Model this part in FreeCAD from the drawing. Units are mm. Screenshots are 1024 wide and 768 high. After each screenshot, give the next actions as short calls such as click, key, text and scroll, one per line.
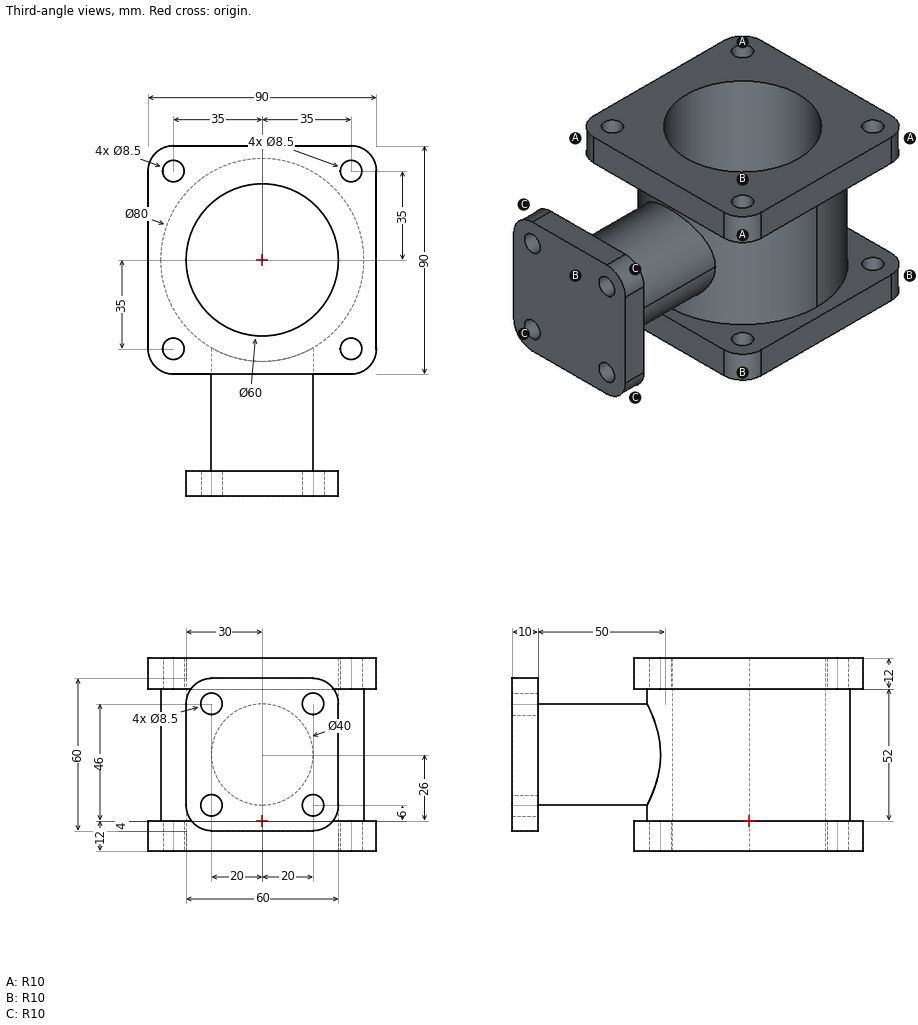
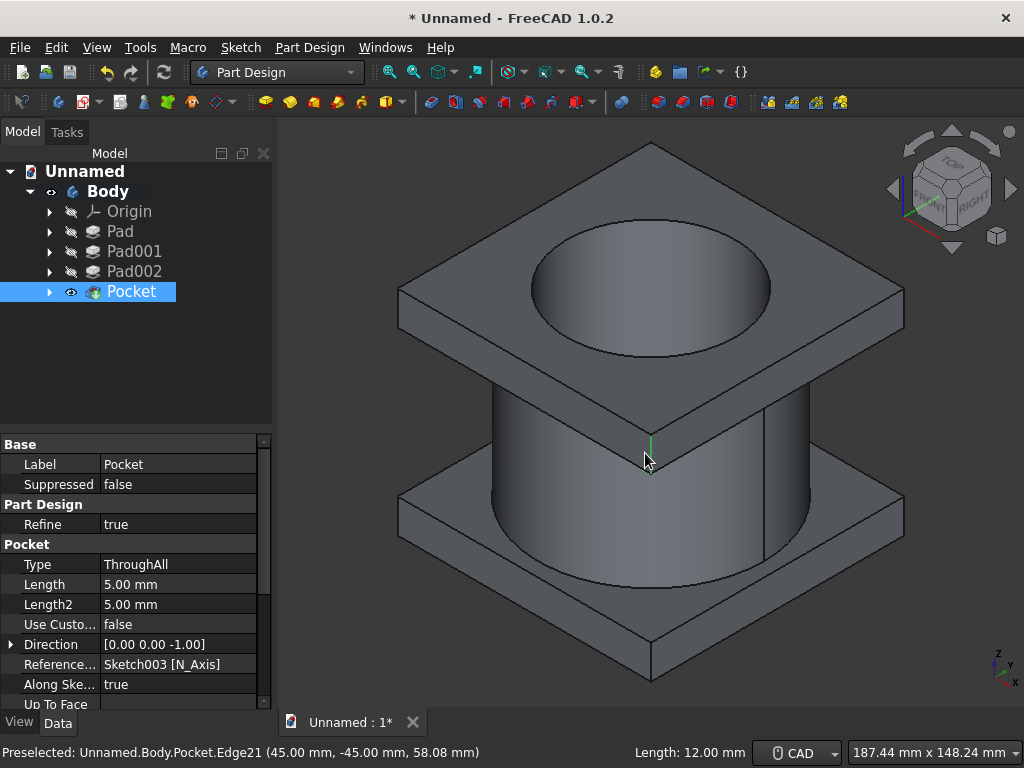
key(1)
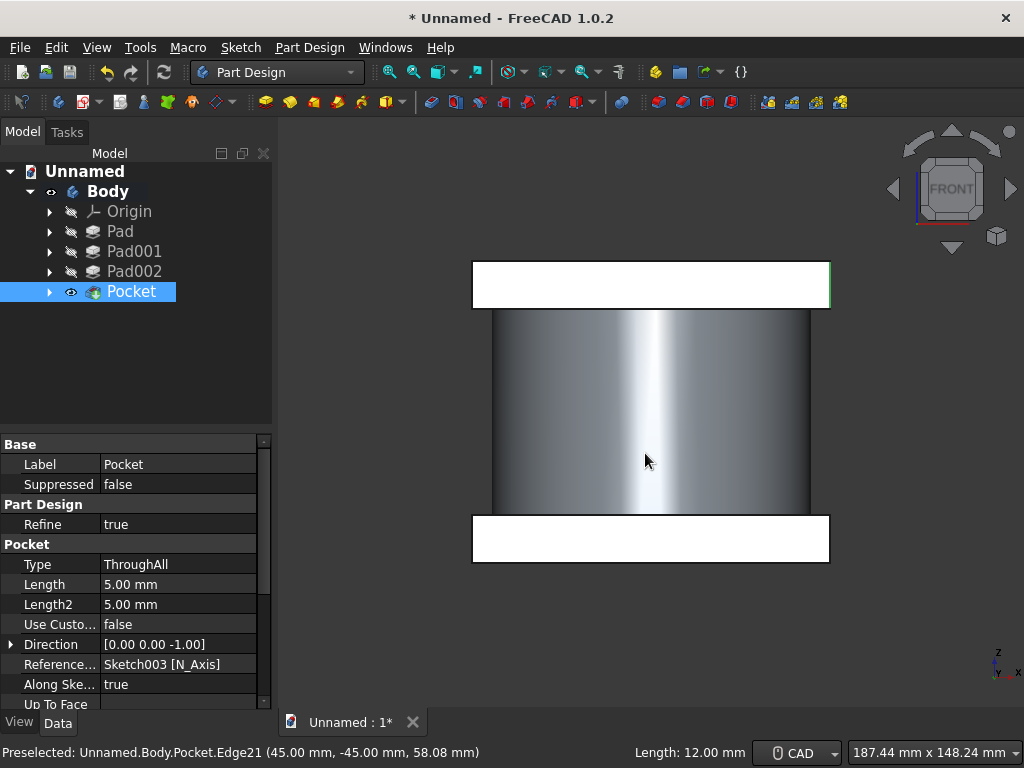
click(472, 284, ctrl)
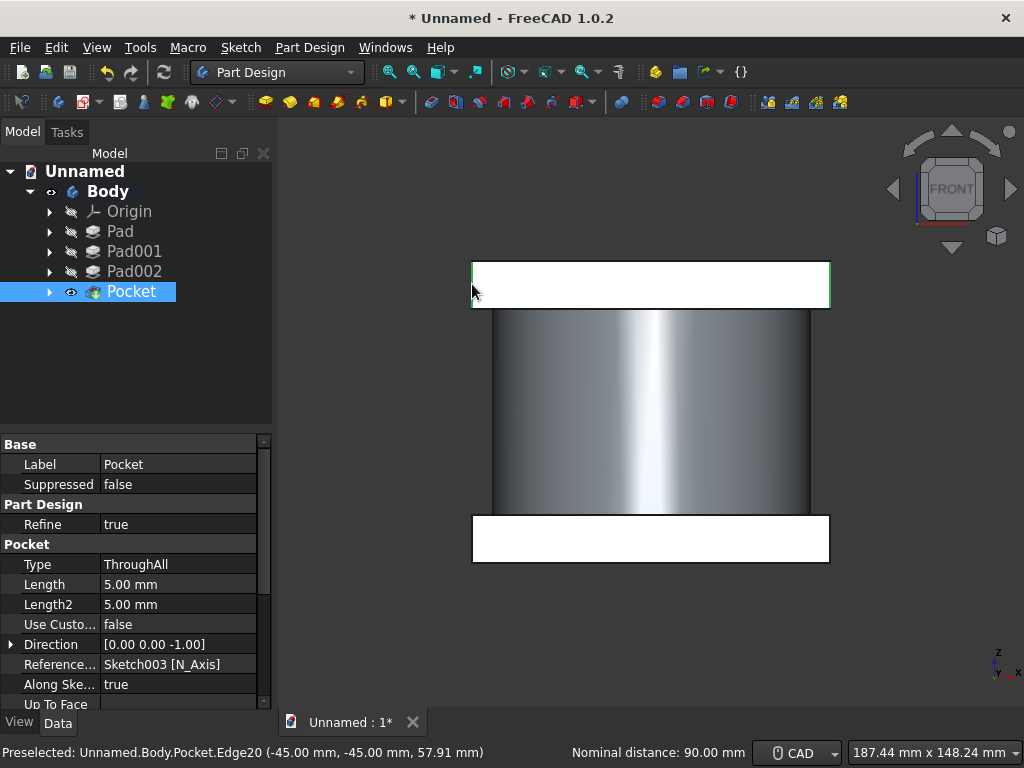
key(3)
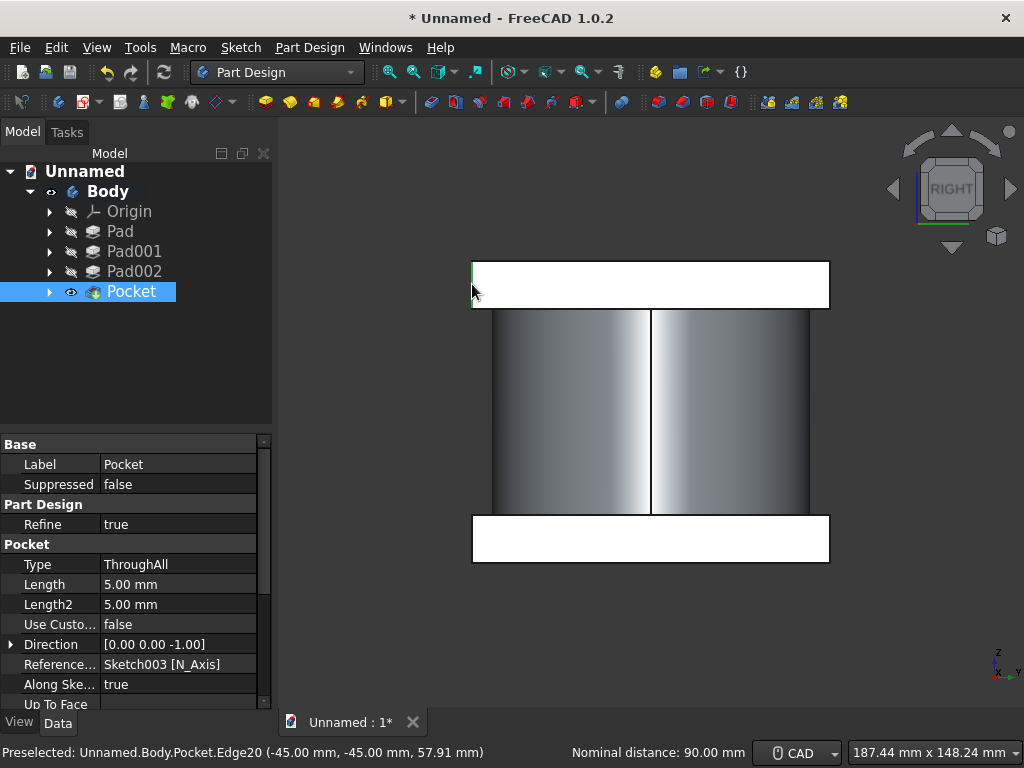
click(830, 284, ctrl)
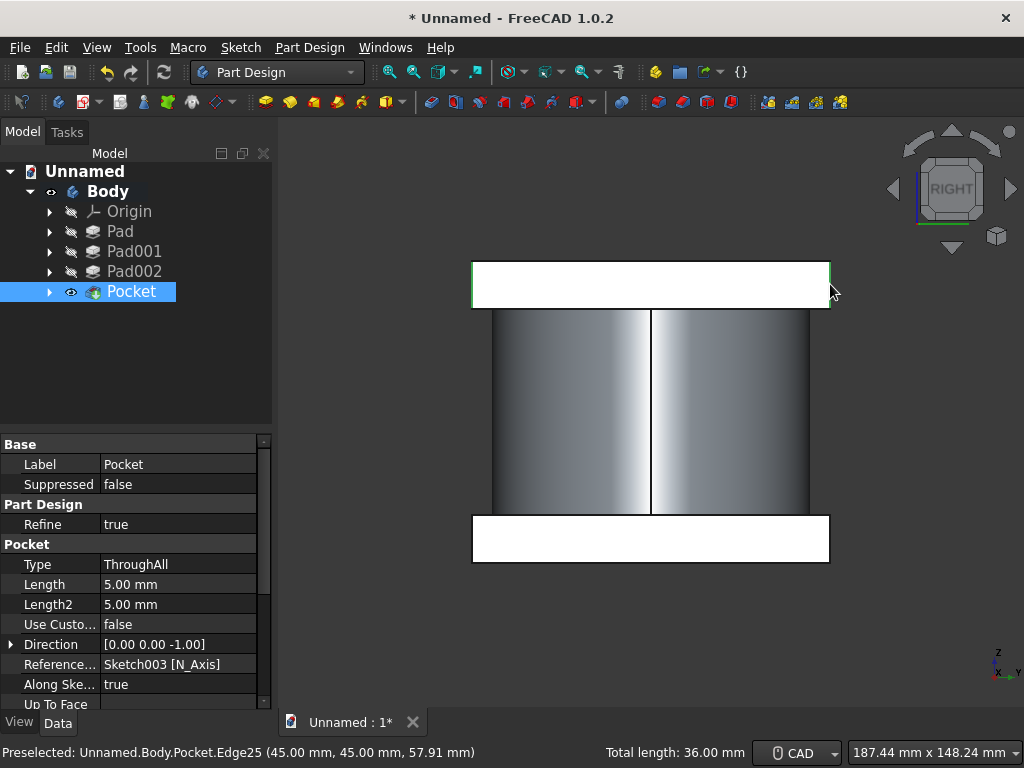
key(5)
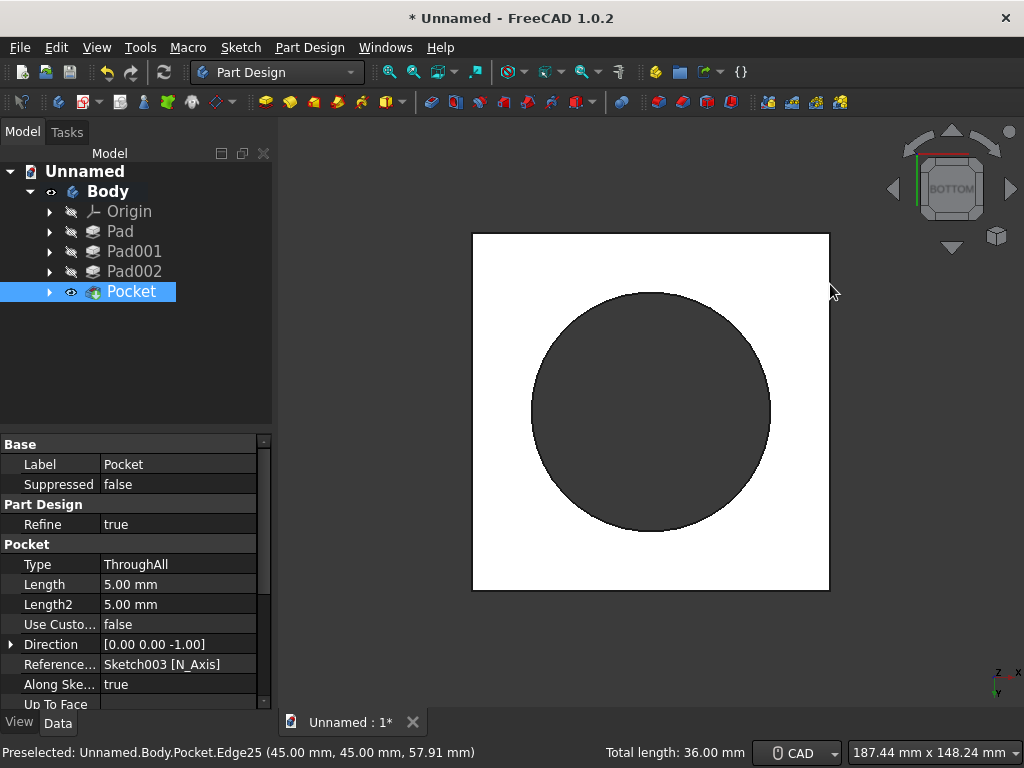
key(4)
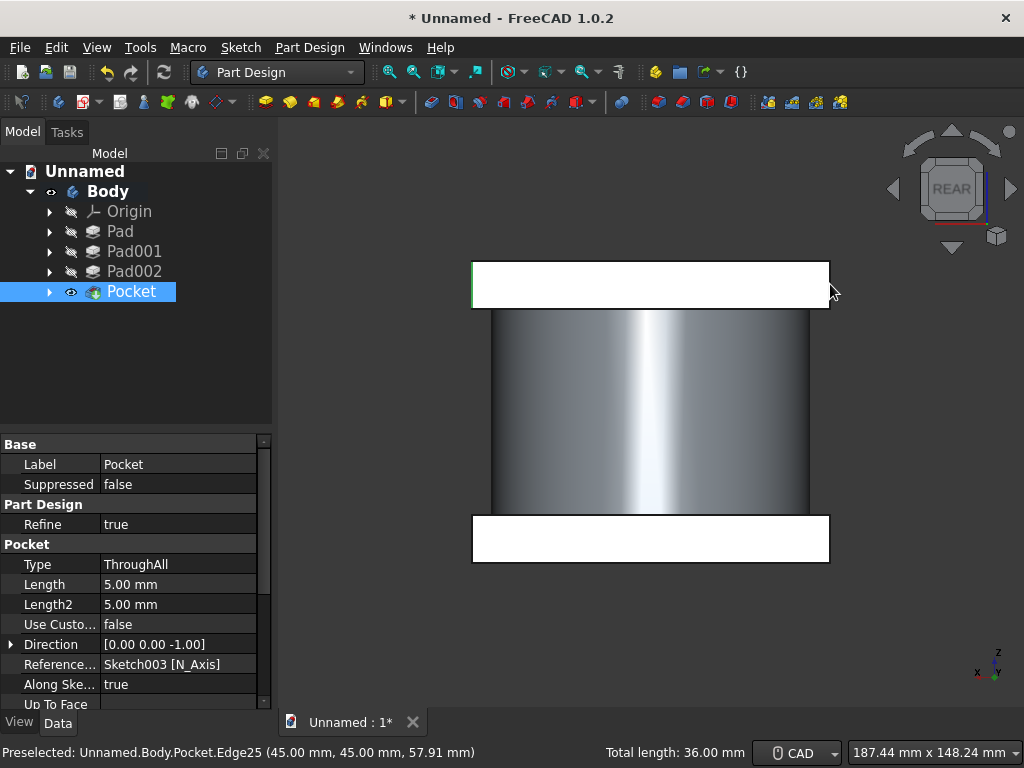
click(830, 284, ctrl)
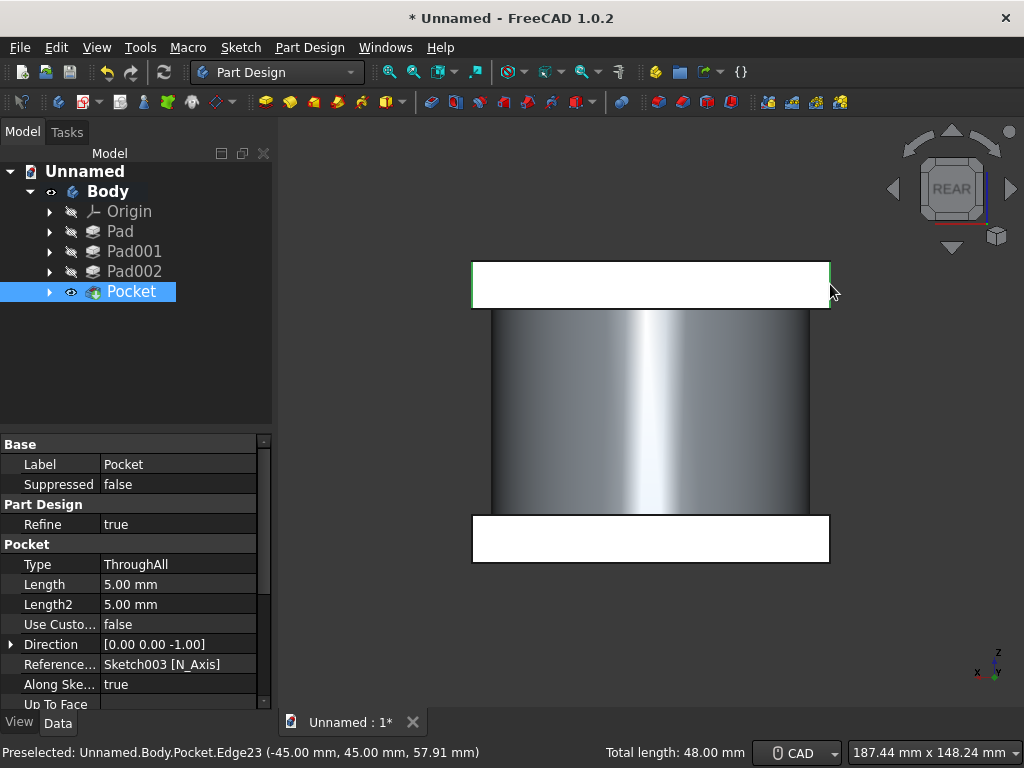
click(660, 102)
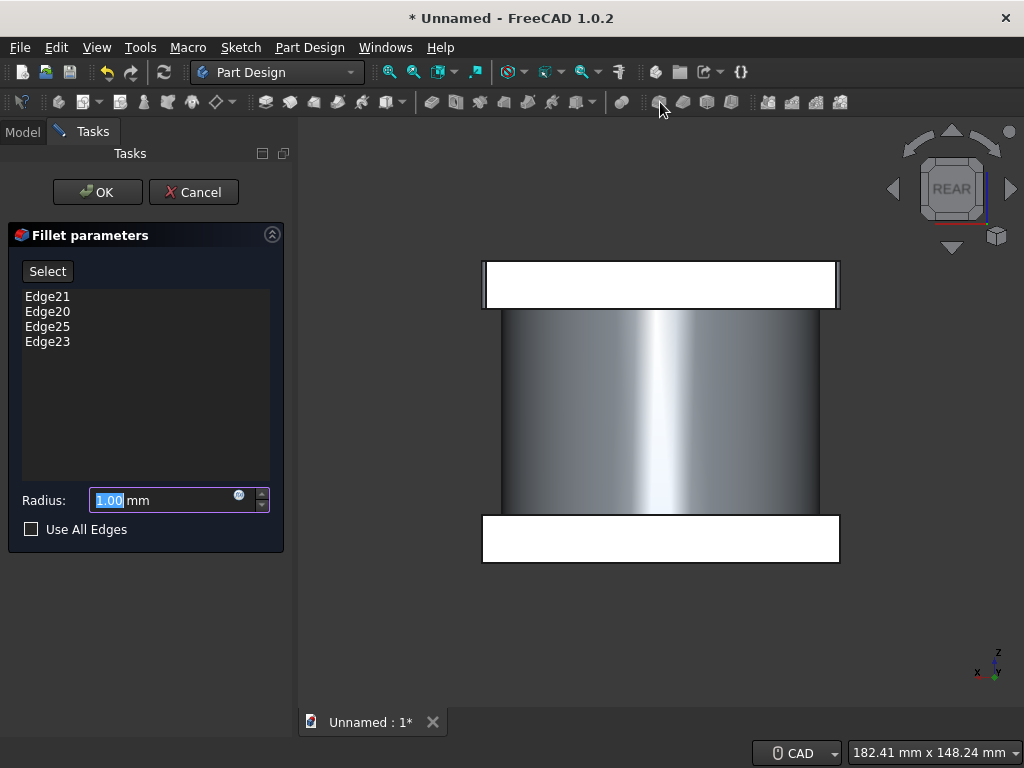
text(10)
key(Tab)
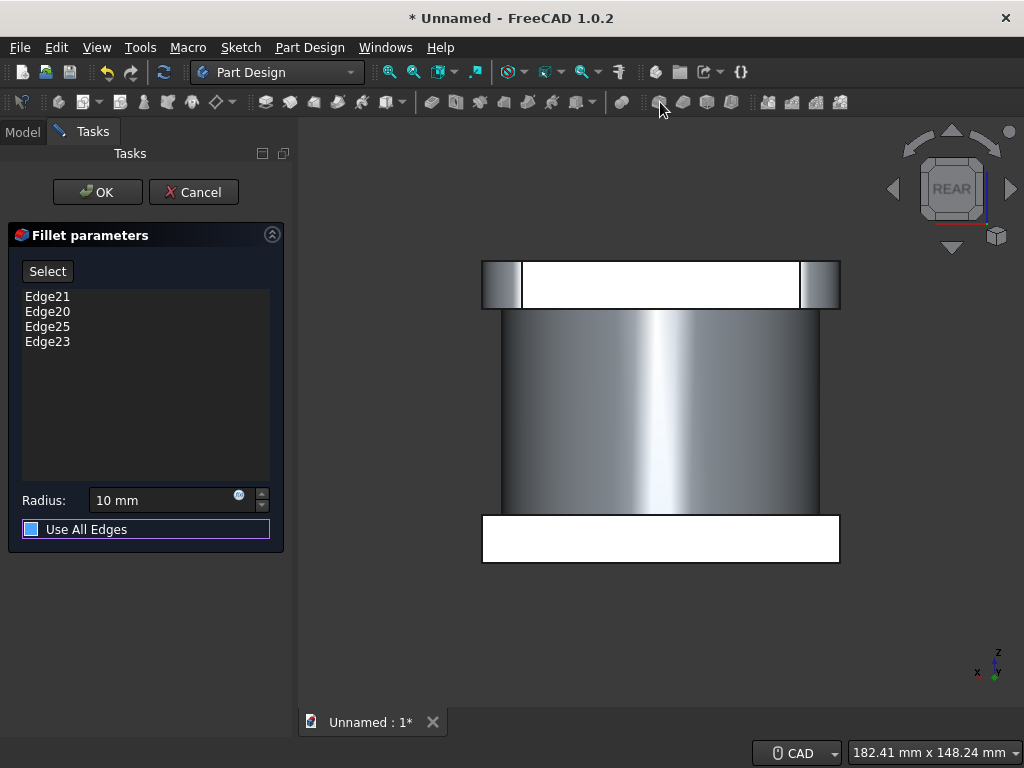
click(98, 192)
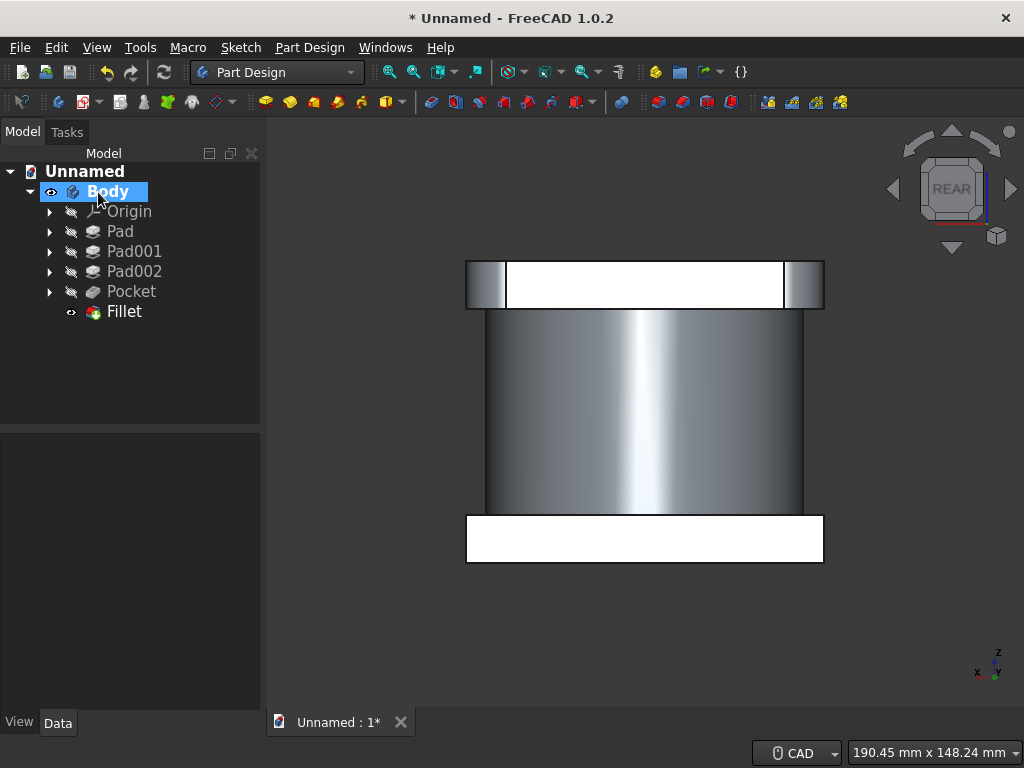
click(824, 538)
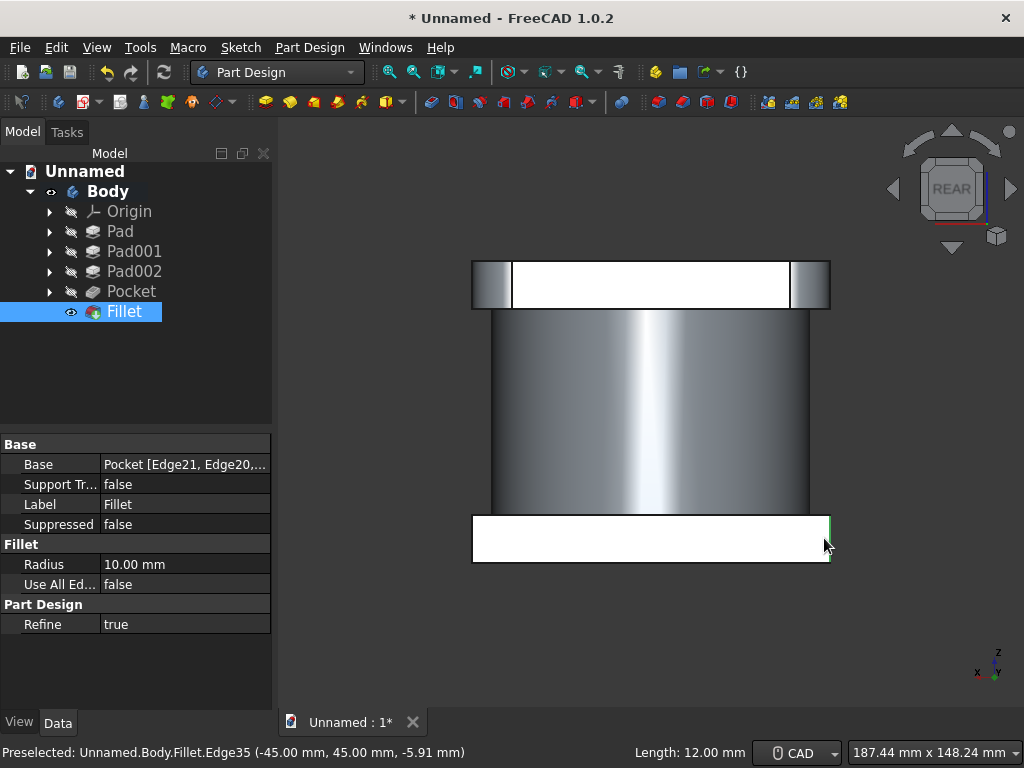
click(472, 538, ctrl)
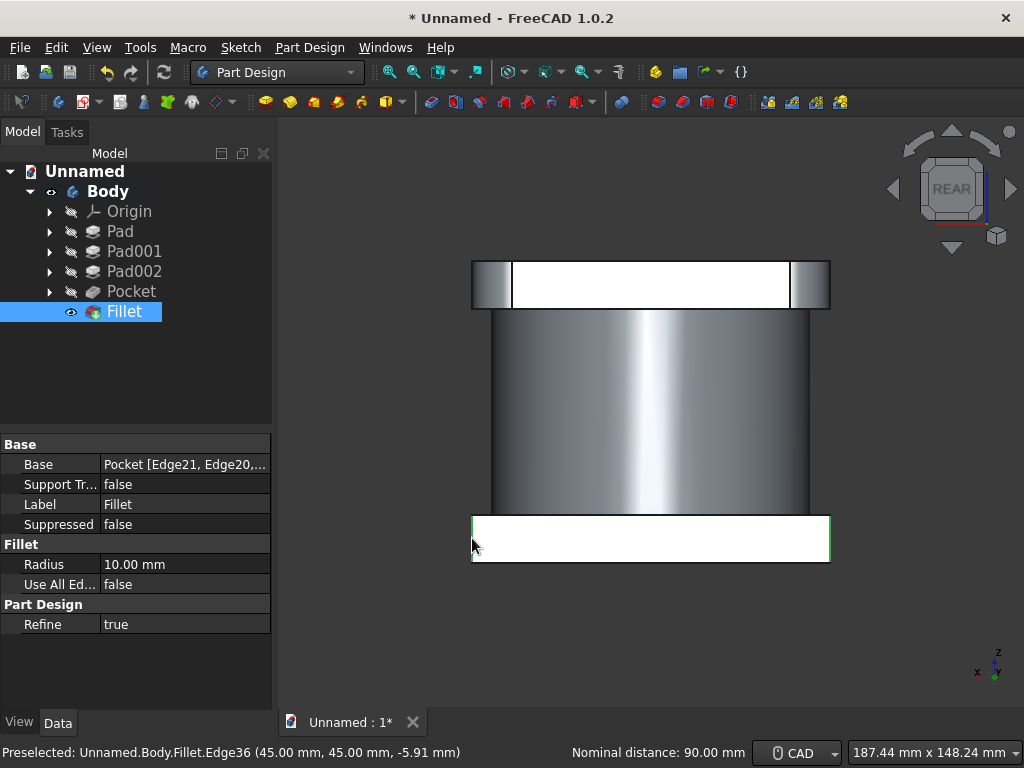
key(0)